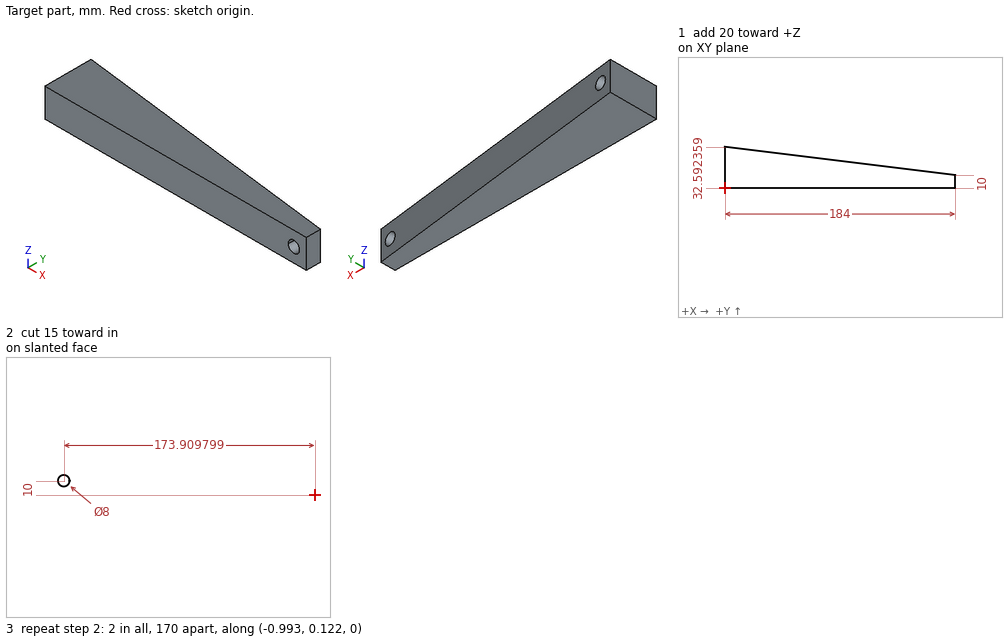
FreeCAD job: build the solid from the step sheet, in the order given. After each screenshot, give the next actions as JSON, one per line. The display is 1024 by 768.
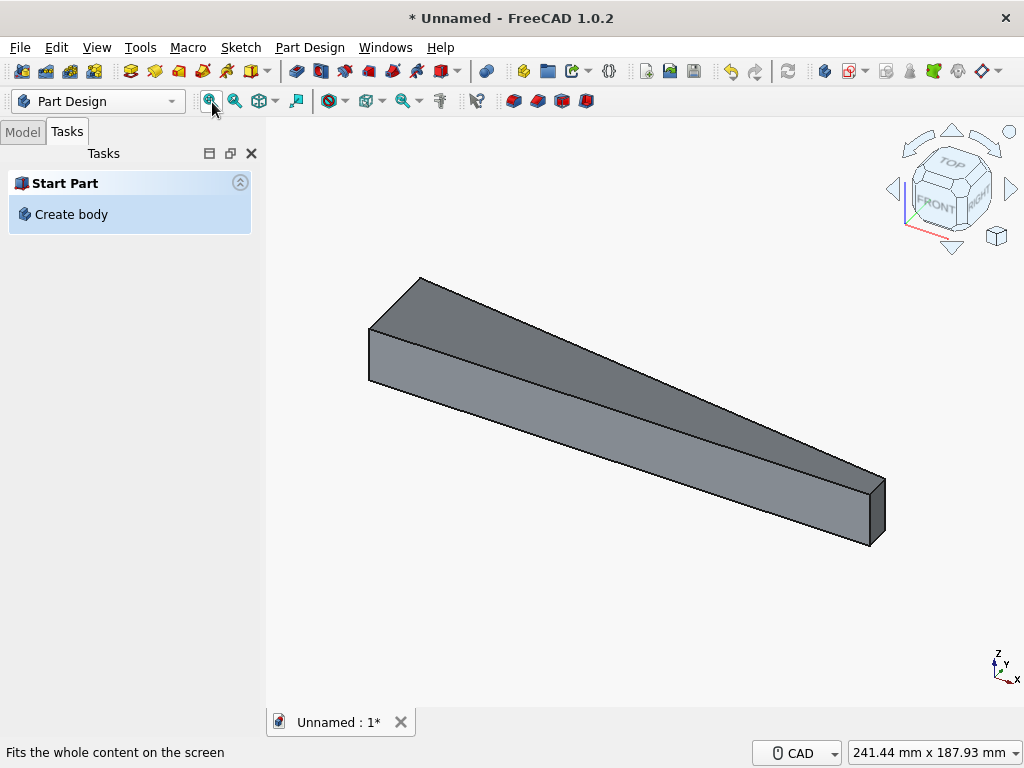
{"action": "key", "text": "4"}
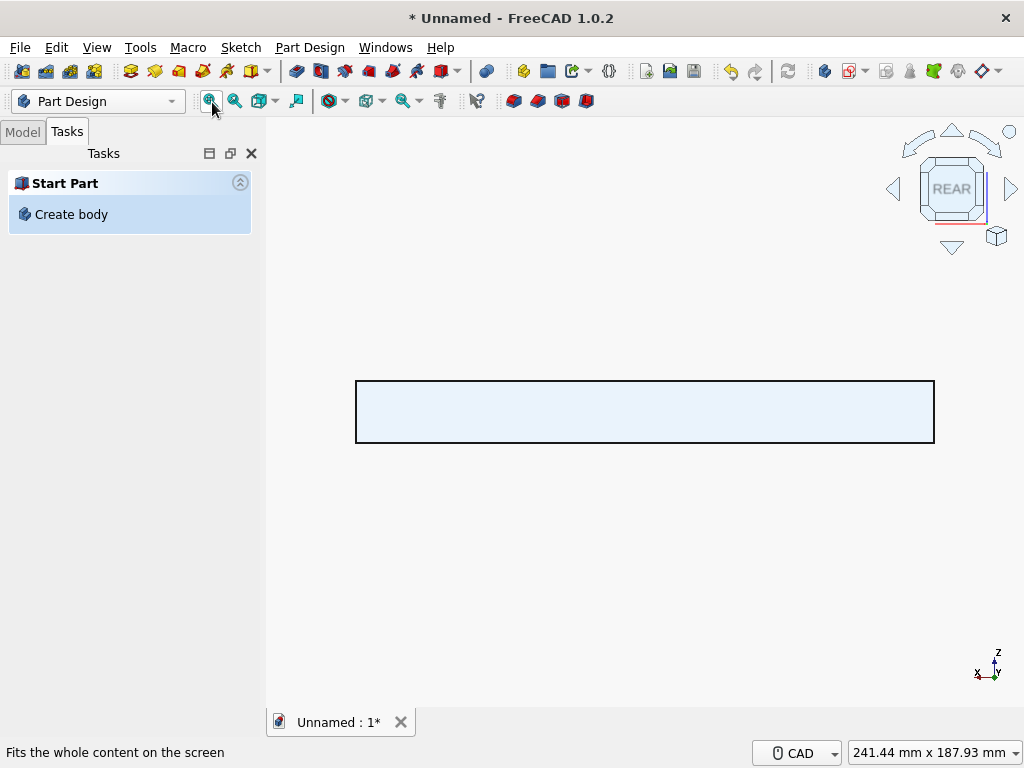
{"action": "left_click", "coordinate": [397, 411]}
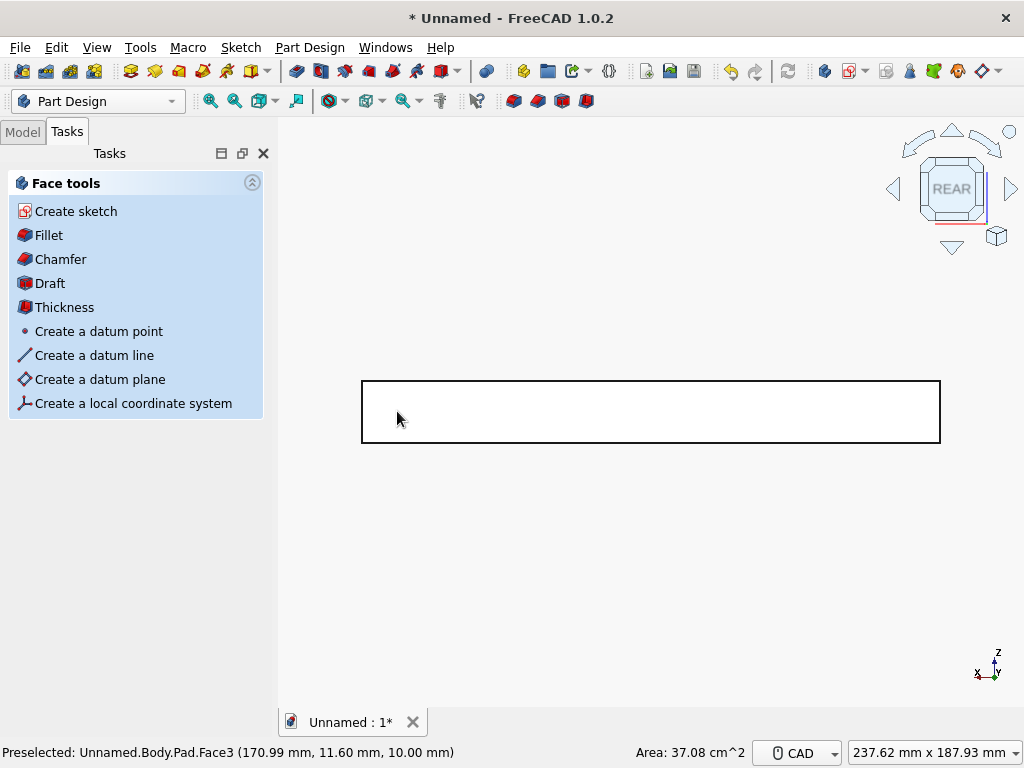
{"action": "left_click", "coordinate": [850, 72]}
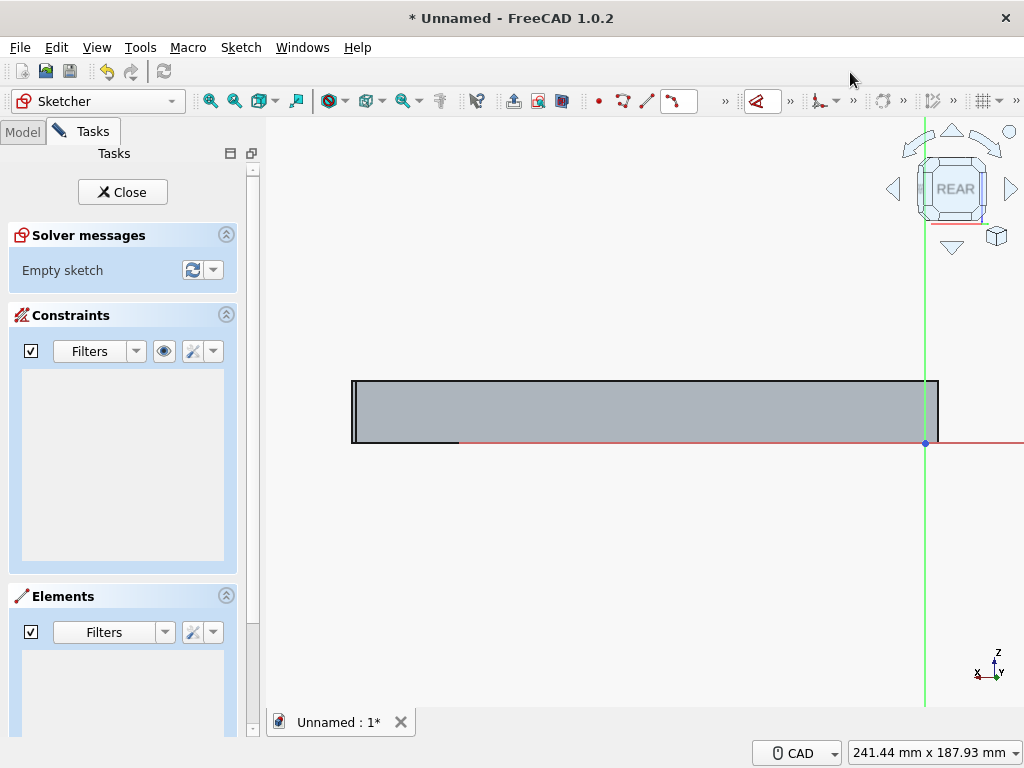
{"action": "left_click", "coordinate": [562, 102]}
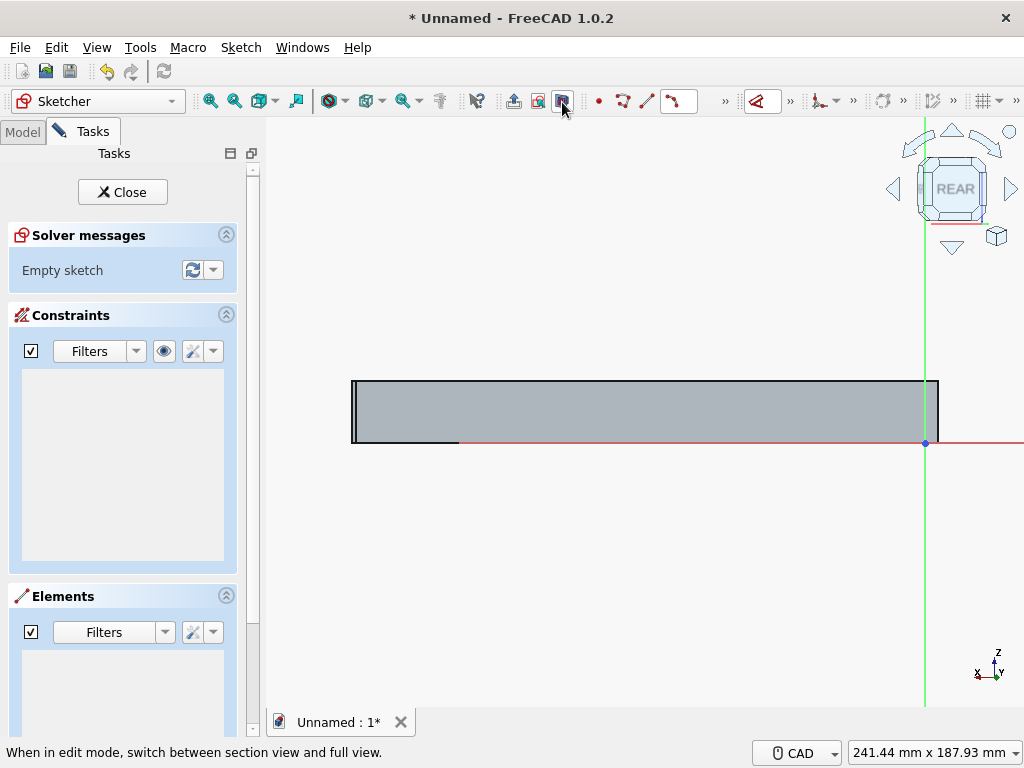
{"action": "scroll", "coordinate": [367, 412], "scroll_direction": "up", "scroll_amount": 14}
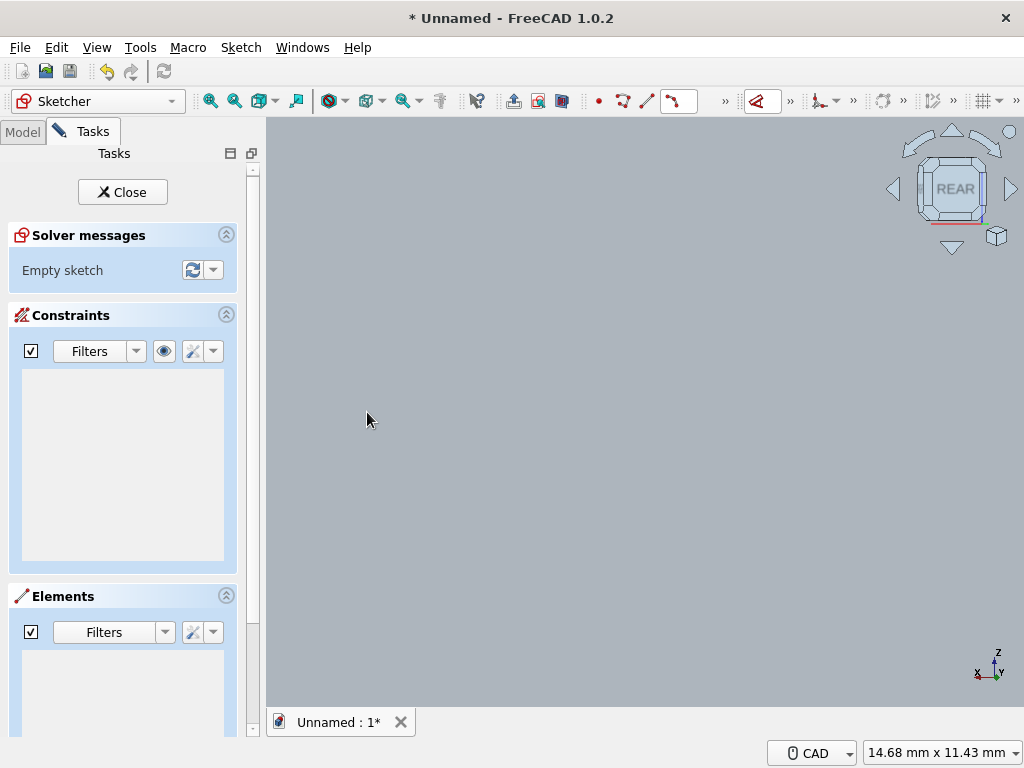
{"action": "key", "text": "g c"}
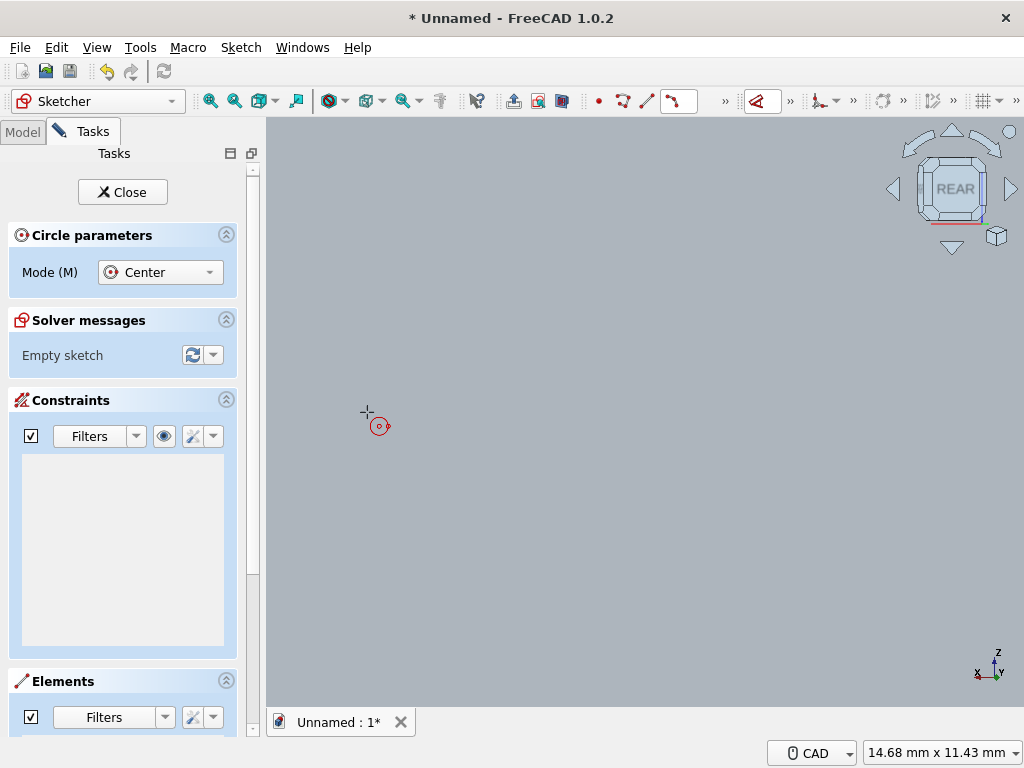
{"action": "left_click", "coordinate": [570, 404]}
{"action": "left_click", "coordinate": [716, 258]}
{"action": "key", "text": "Escape"}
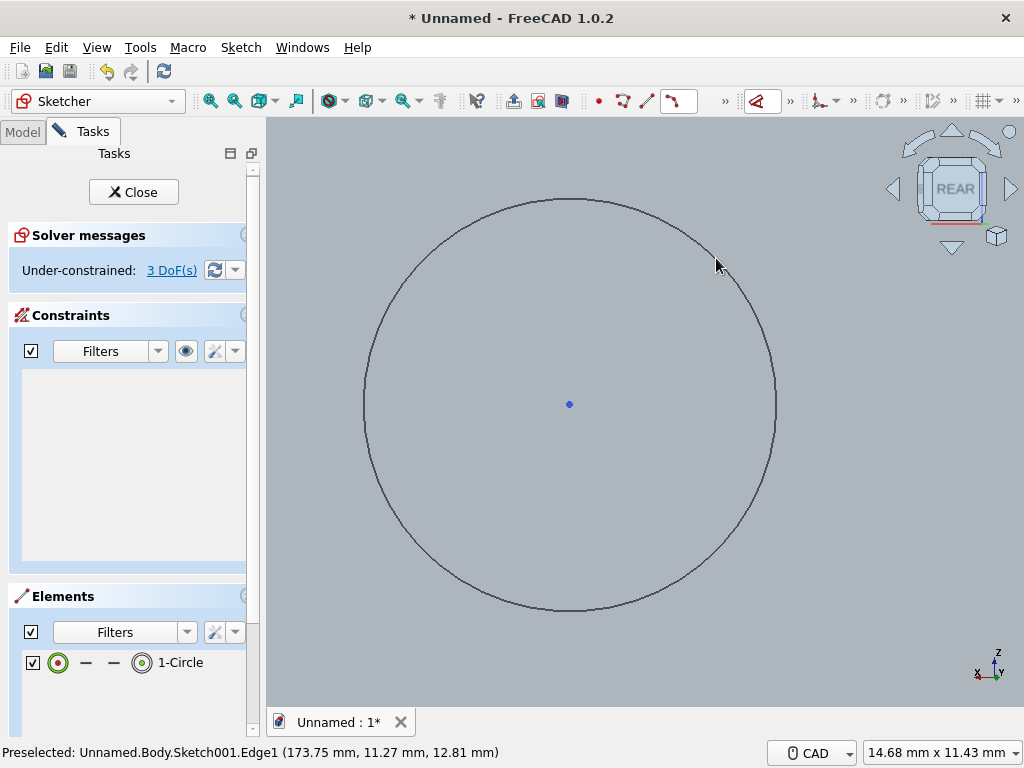
{"action": "left_click", "coordinate": [716, 259]}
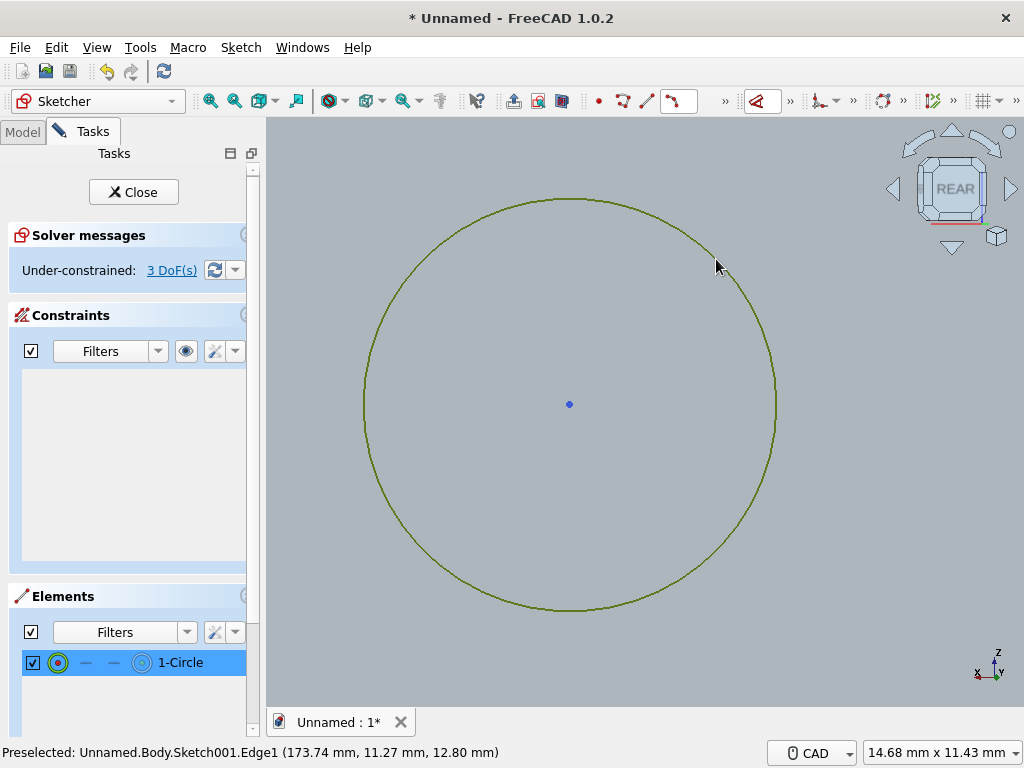
{"action": "key", "text": "k o"}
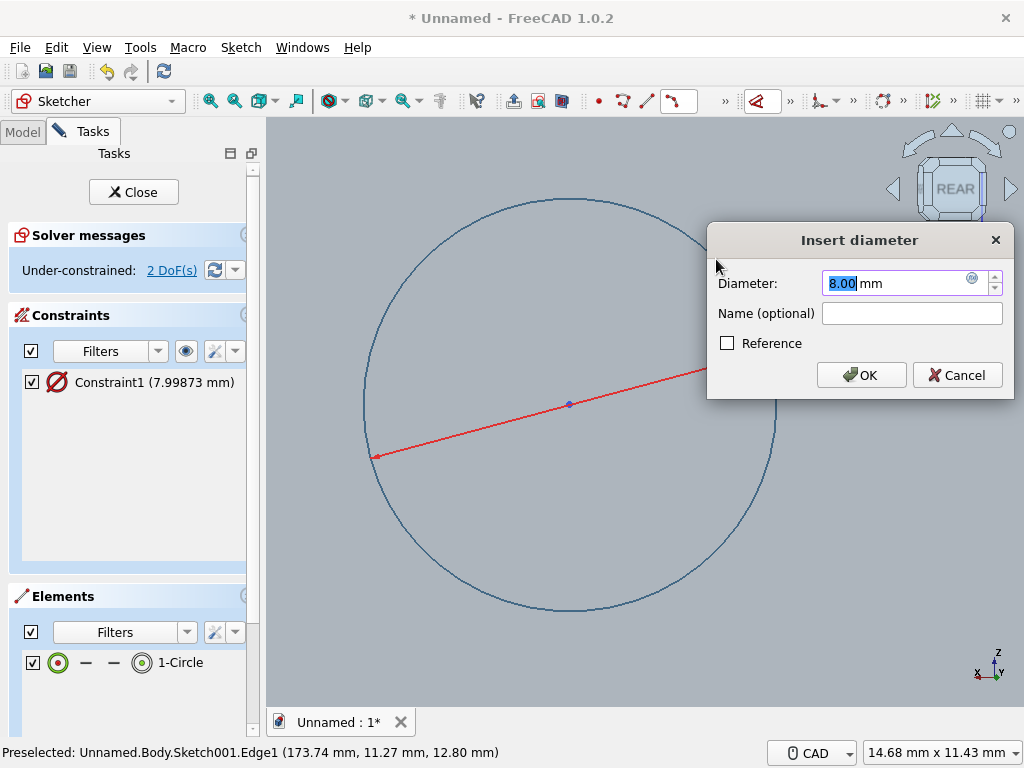
{"action": "type", "text": "8"}
{"action": "key", "text": "Return"}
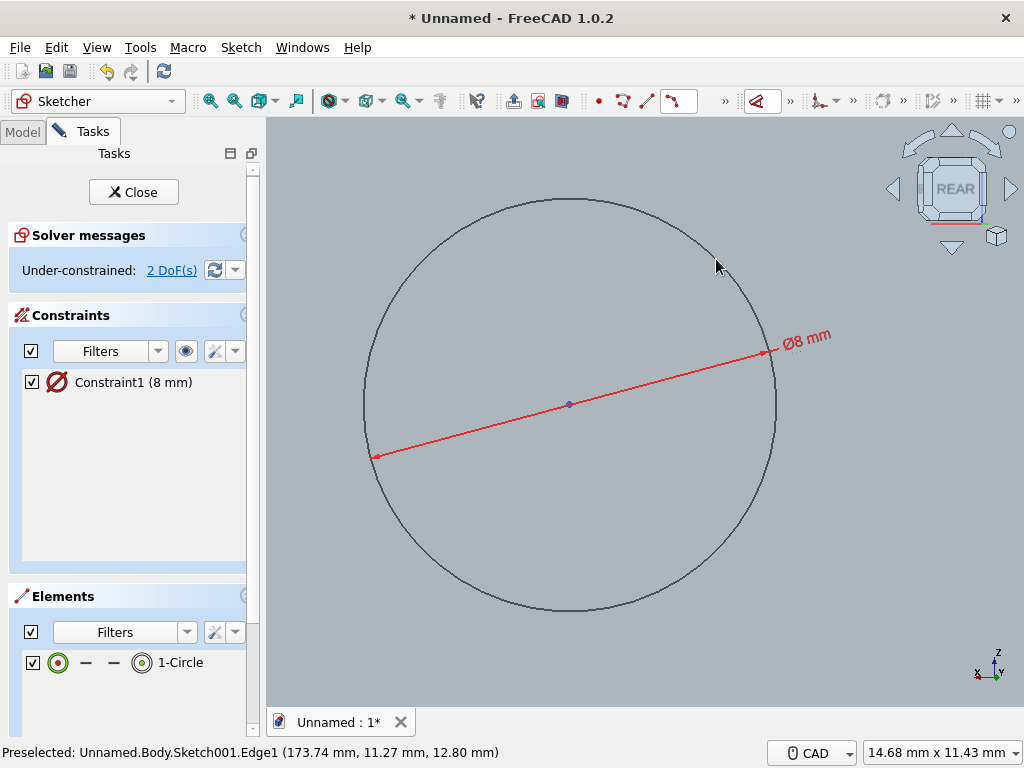
{"action": "left_click", "coordinate": [570, 405]}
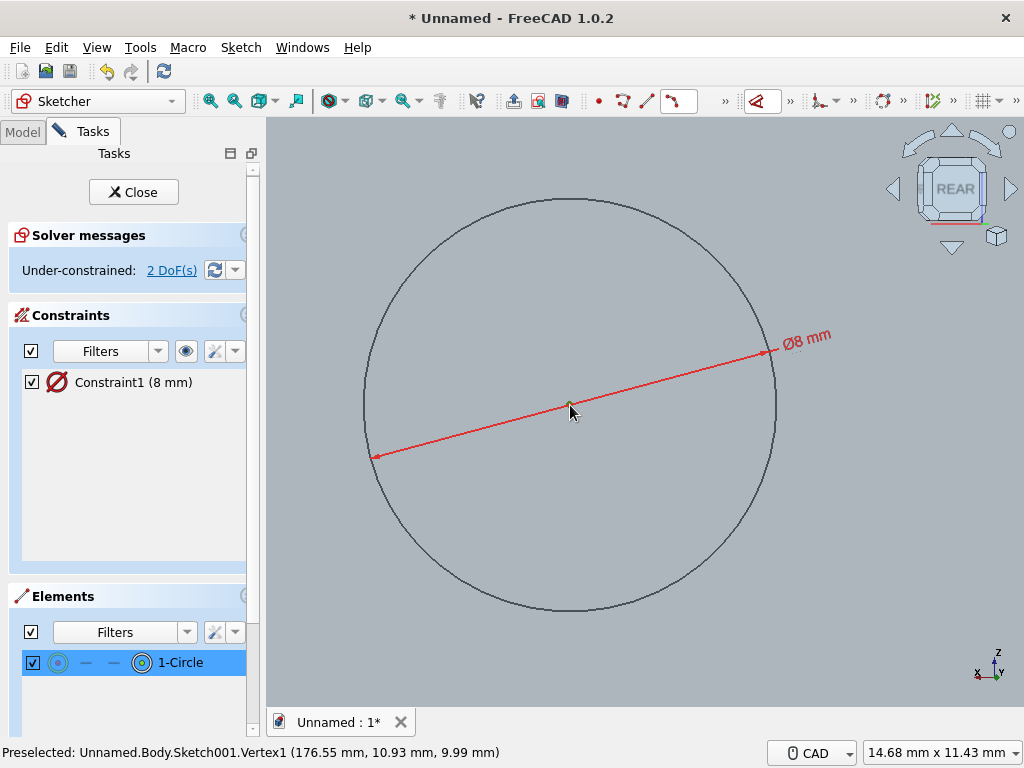
{"action": "left_click", "coordinate": [776, 102]}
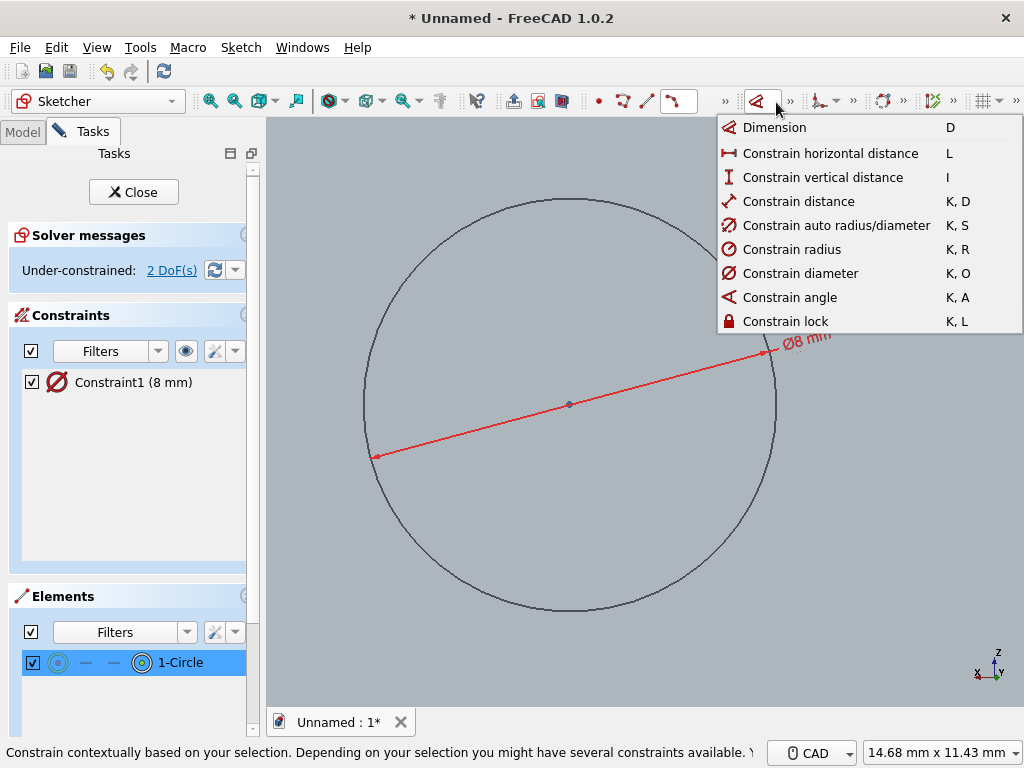
{"action": "left_click", "coordinate": [870, 177]}